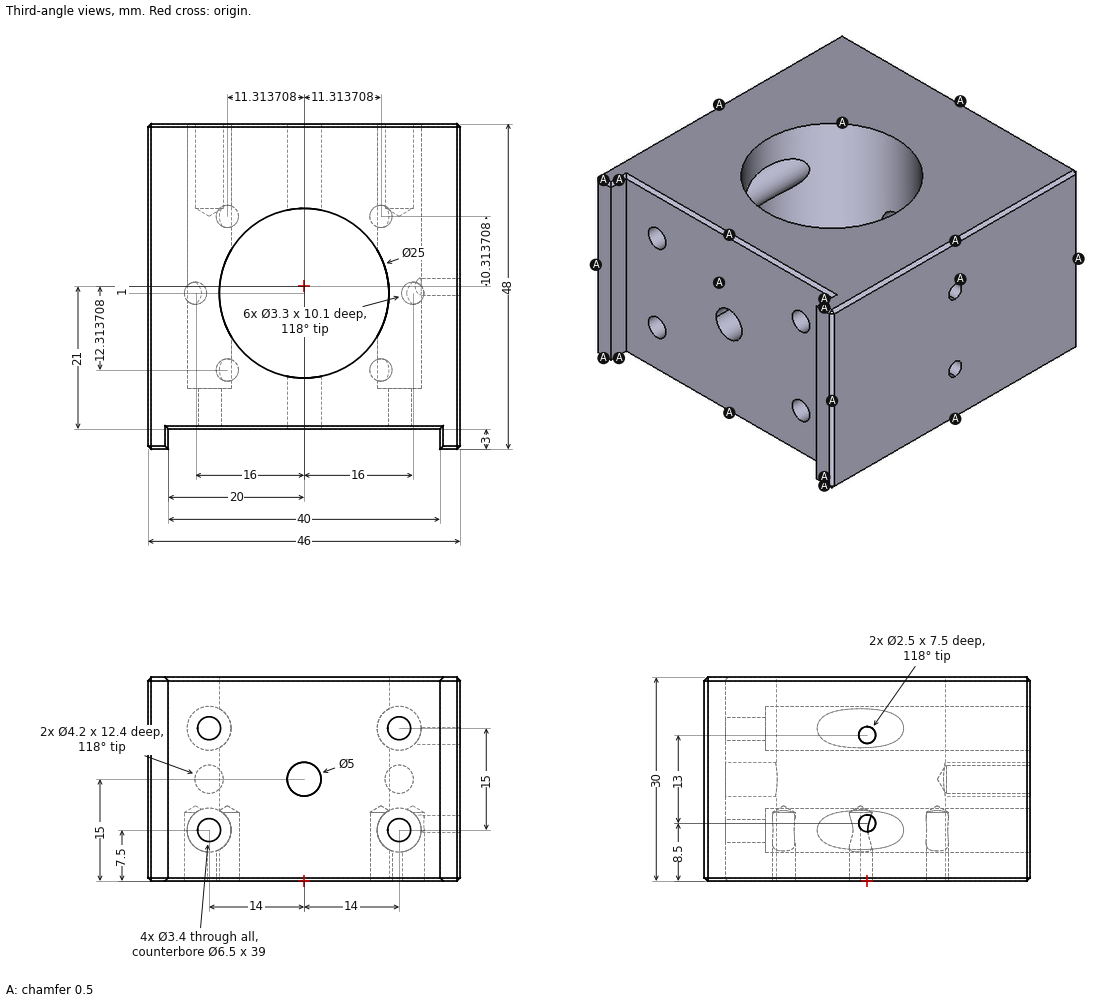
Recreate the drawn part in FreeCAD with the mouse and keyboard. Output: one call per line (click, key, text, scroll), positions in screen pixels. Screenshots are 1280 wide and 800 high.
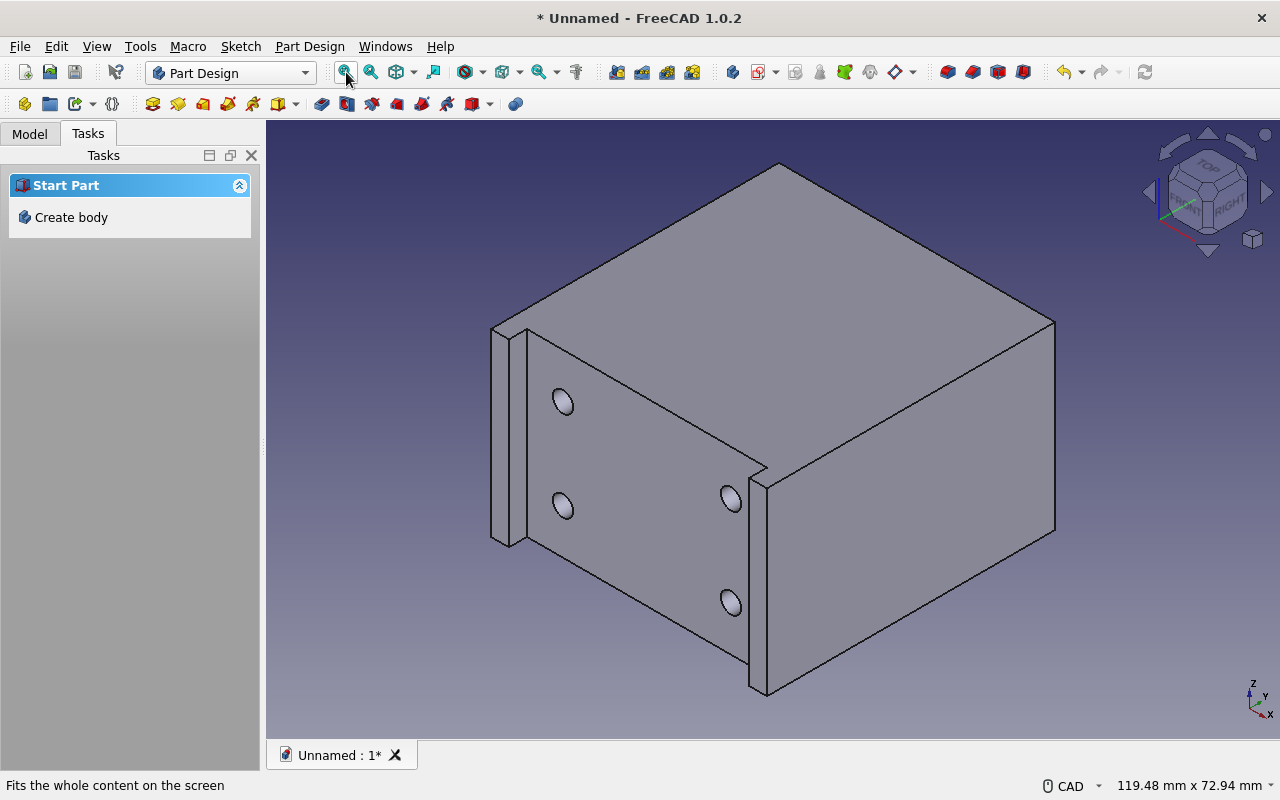
click(773, 325)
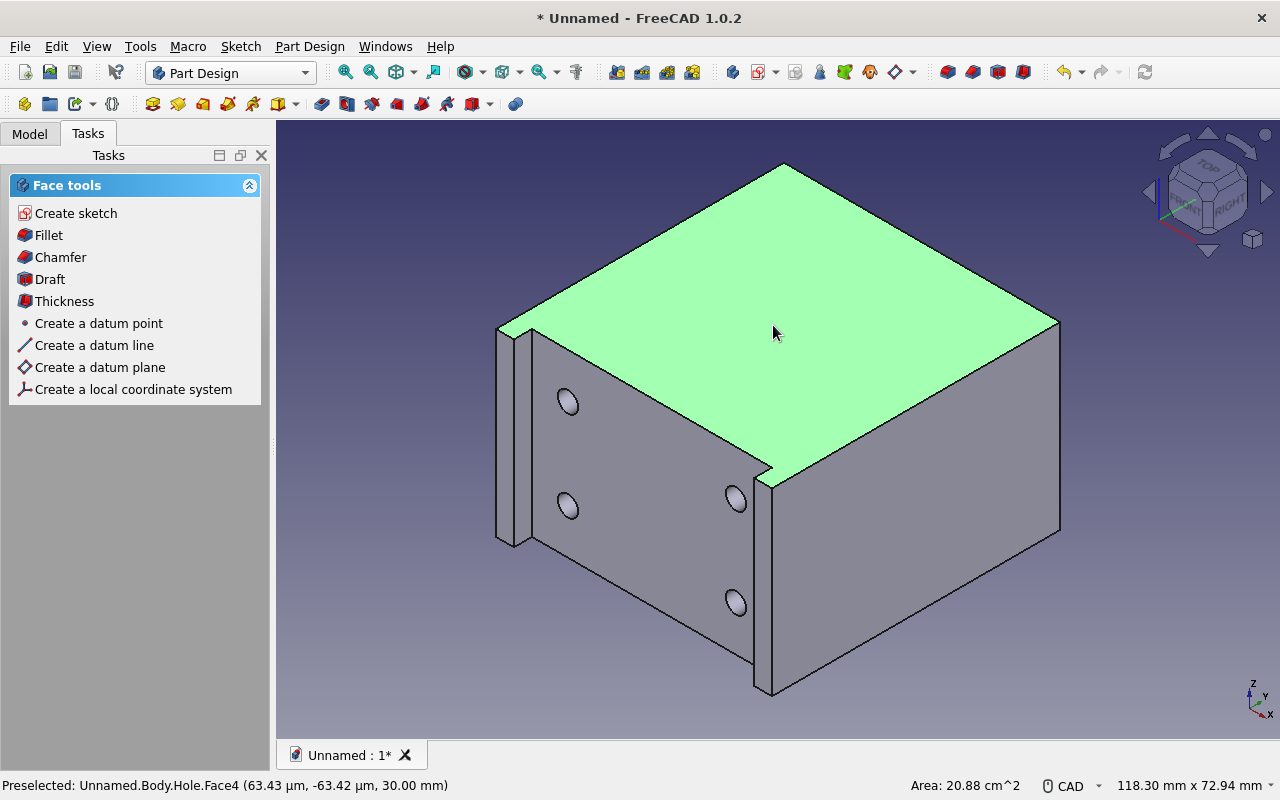
click(758, 72)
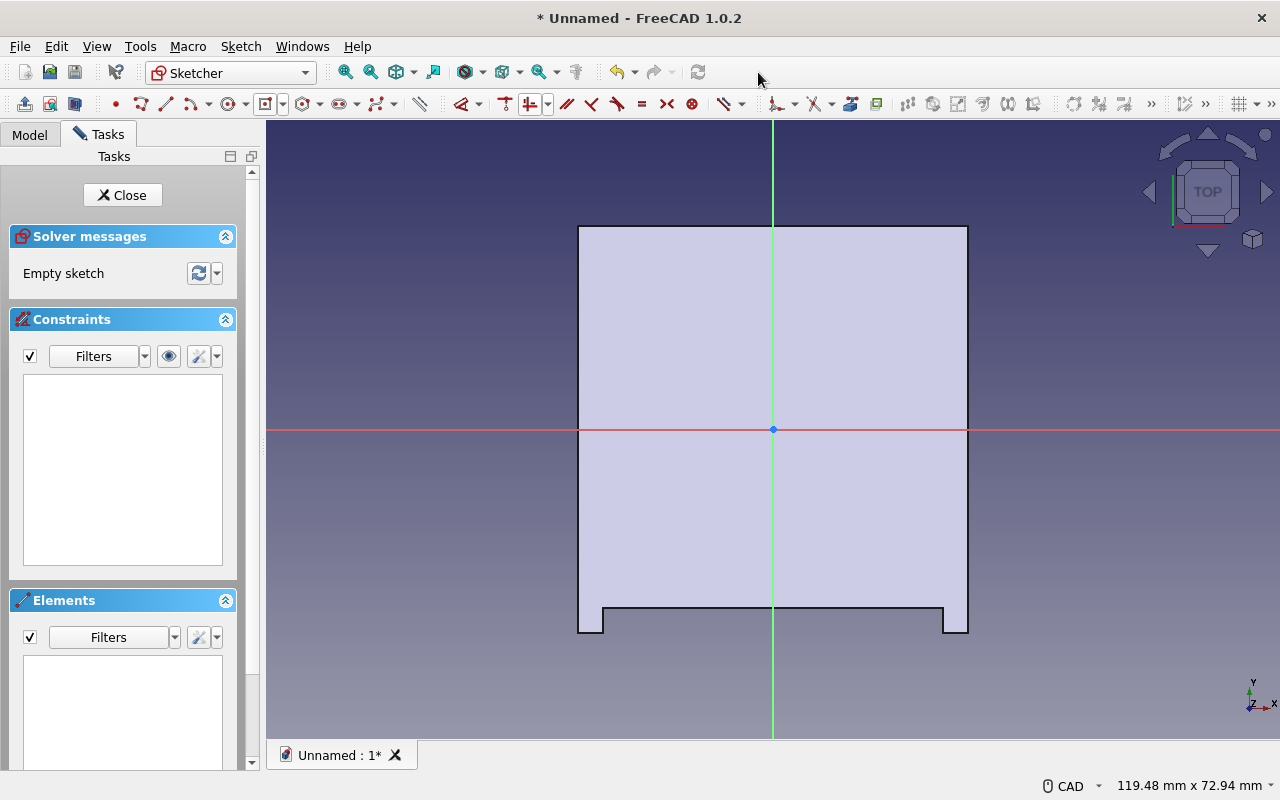
scroll(856, 448, up, 3)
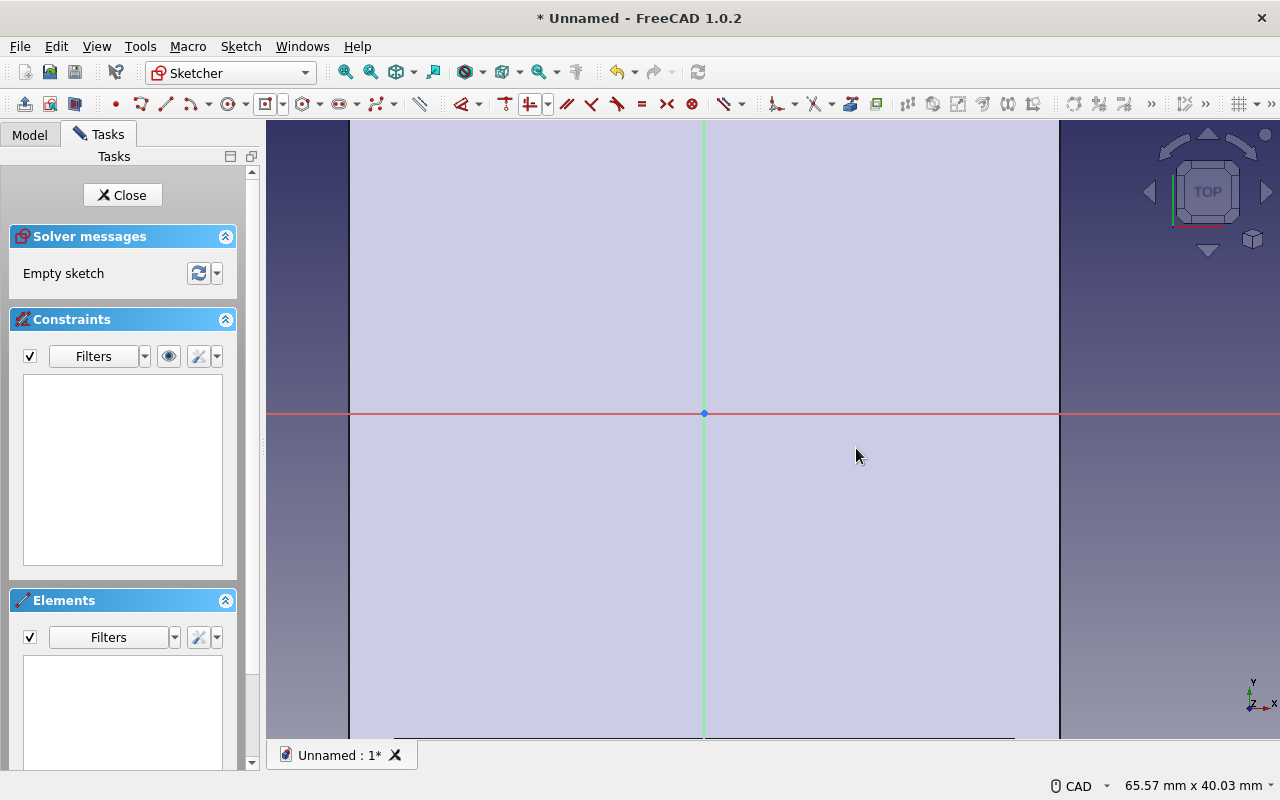
click(228, 104)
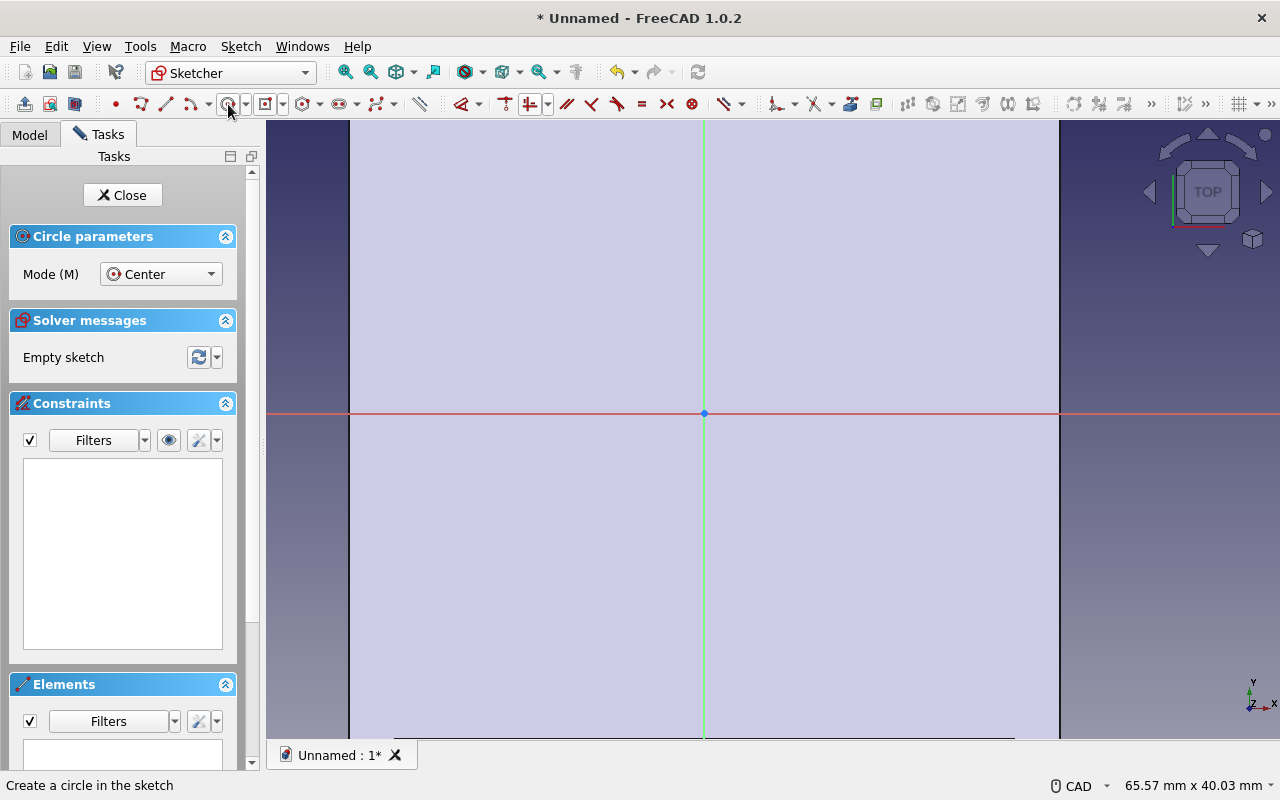
click(704, 429)
move(841, 293)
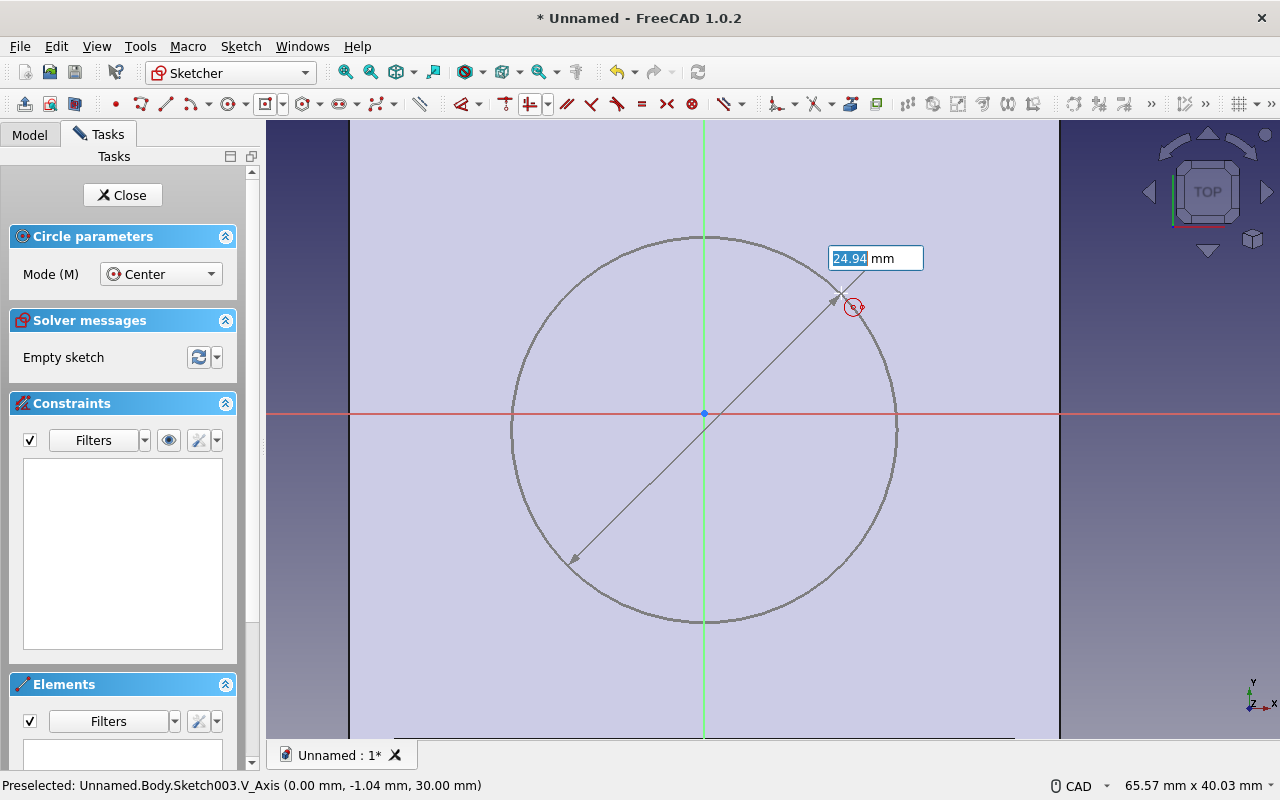
text(25)
key(Return)
key(Escape)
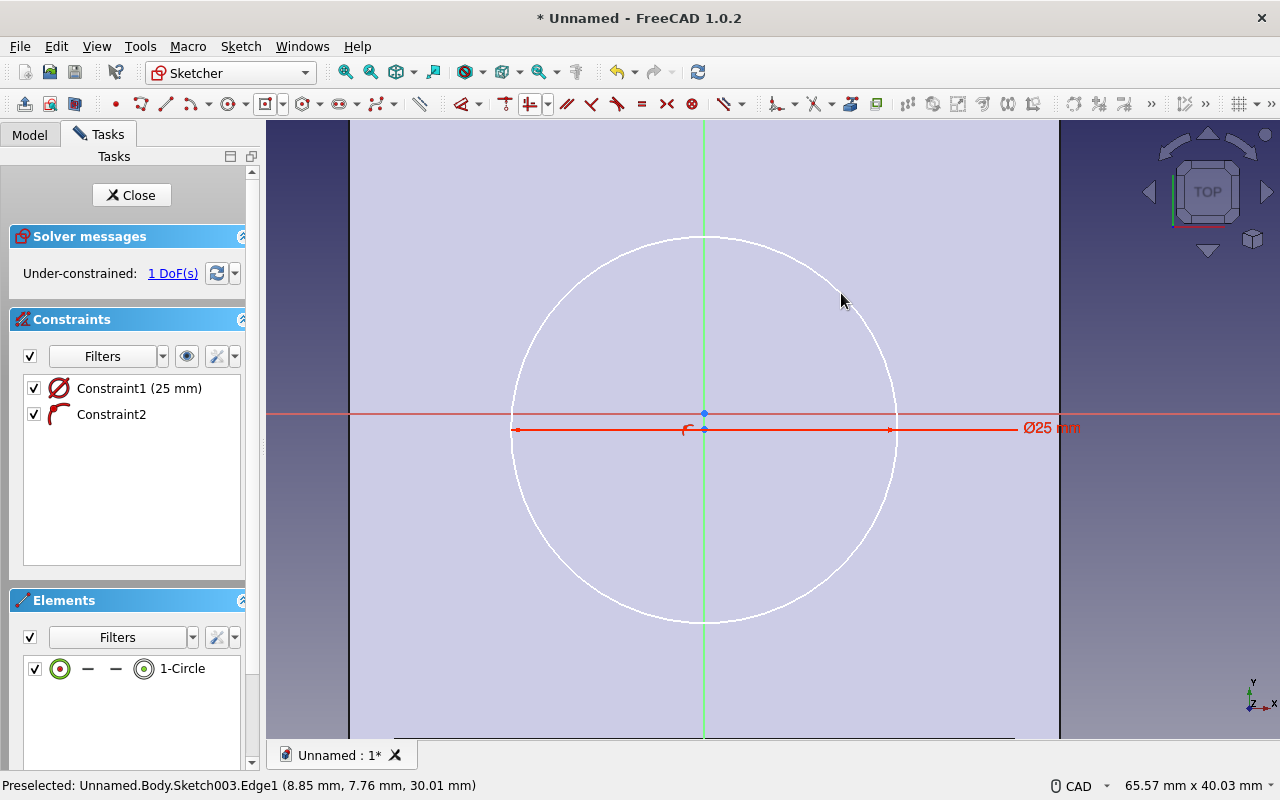
click(460, 104)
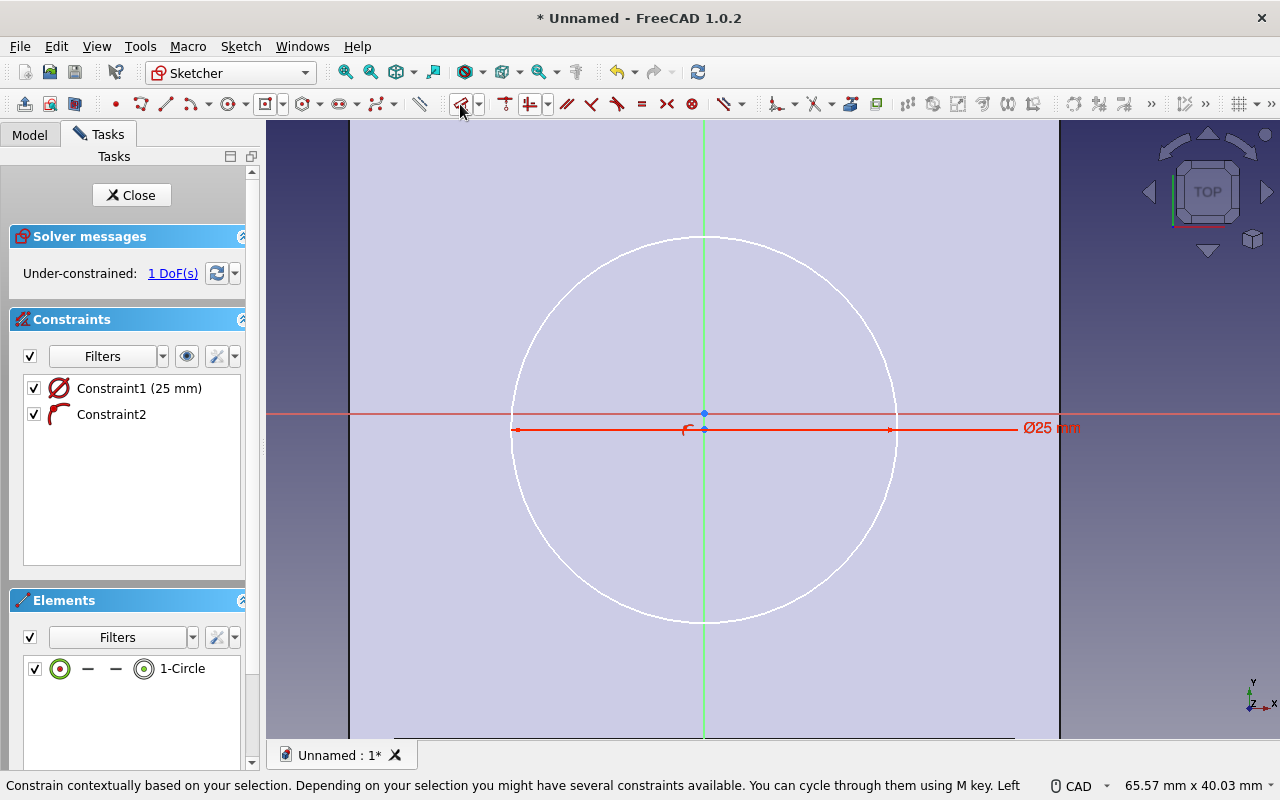
scroll(704, 430, up, 5)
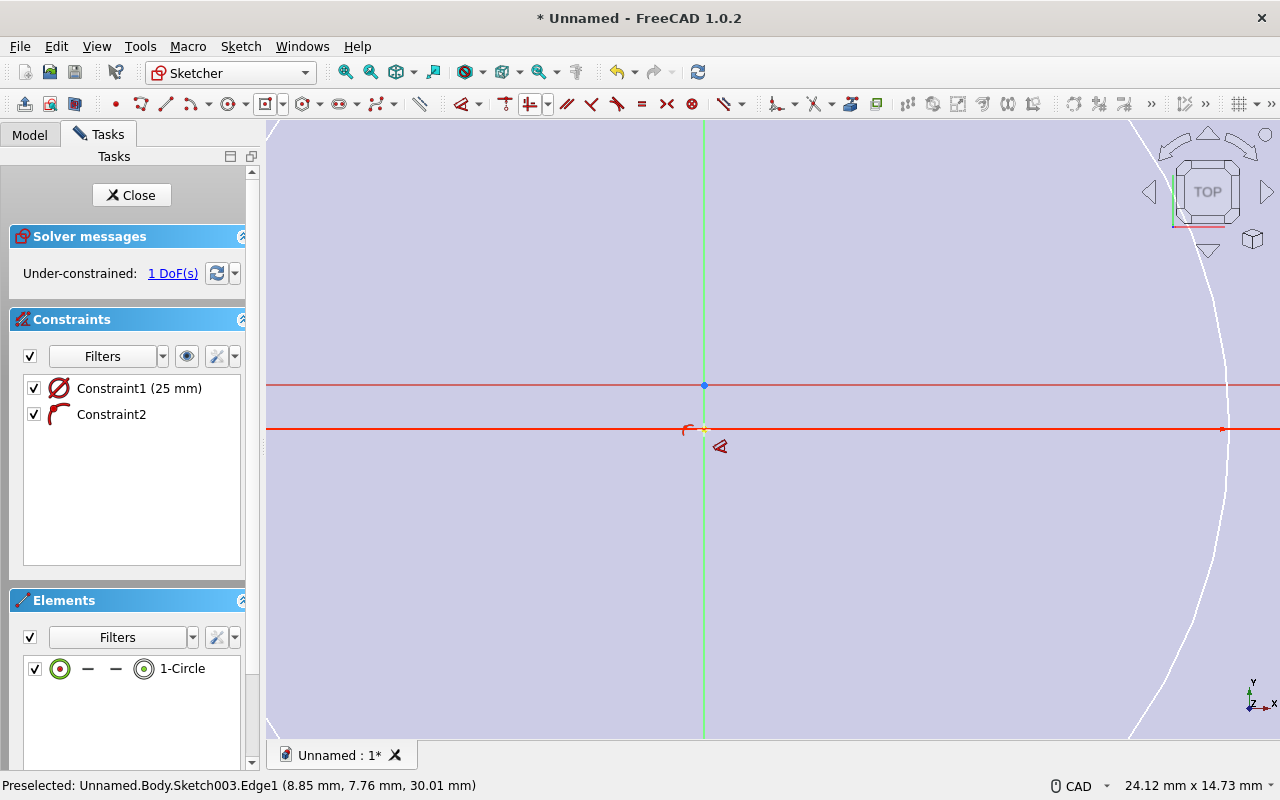
click(704, 429)
click(738, 407)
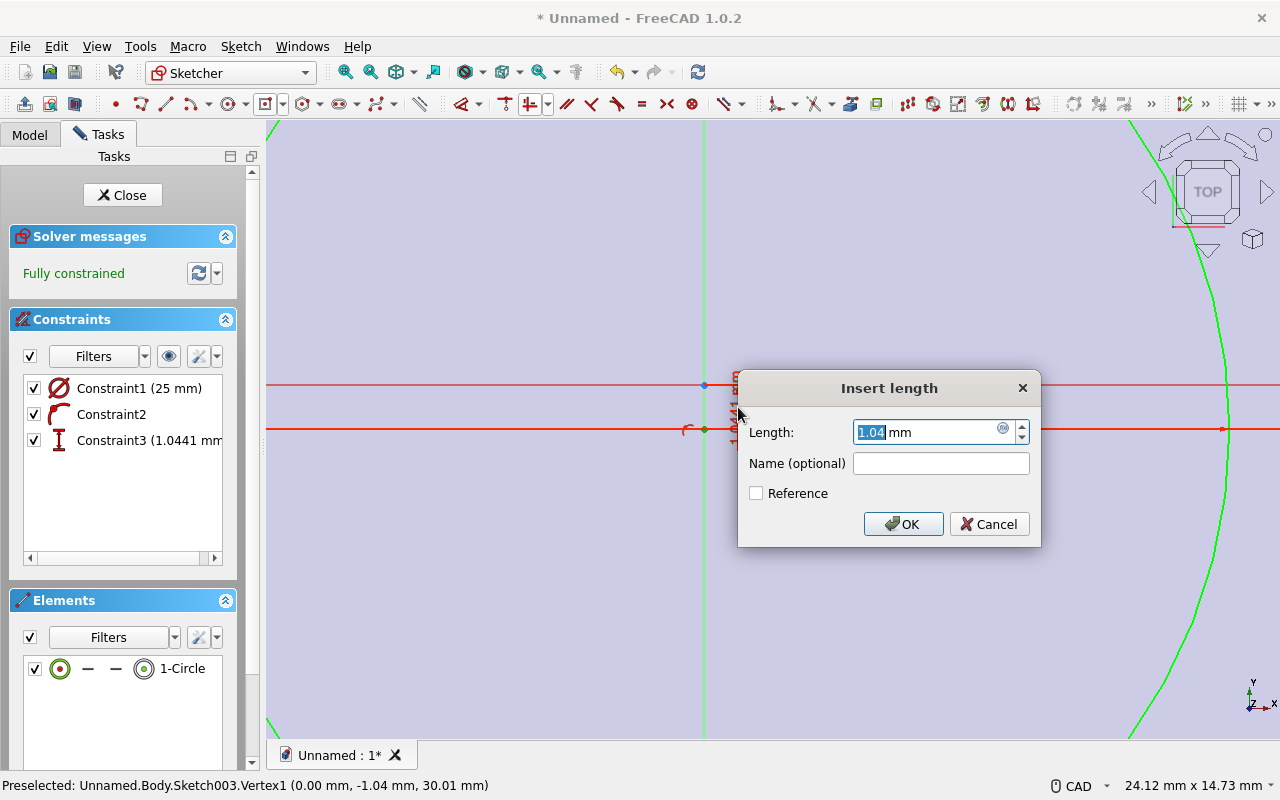
text(1)
key(Return)
key(Escape)